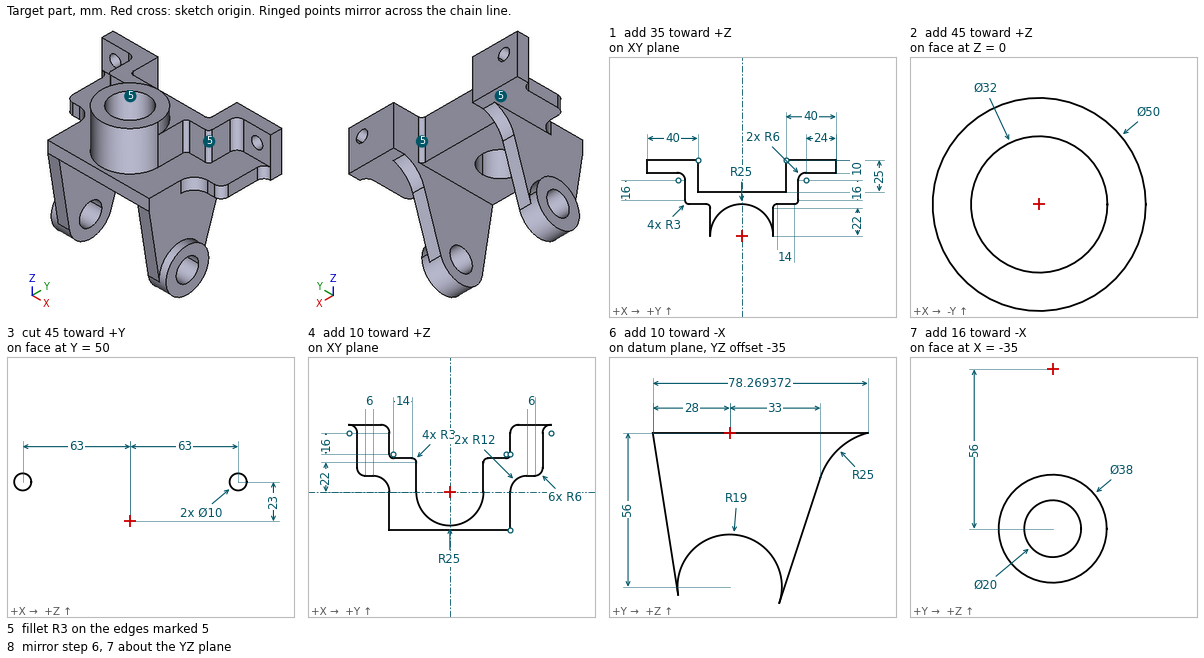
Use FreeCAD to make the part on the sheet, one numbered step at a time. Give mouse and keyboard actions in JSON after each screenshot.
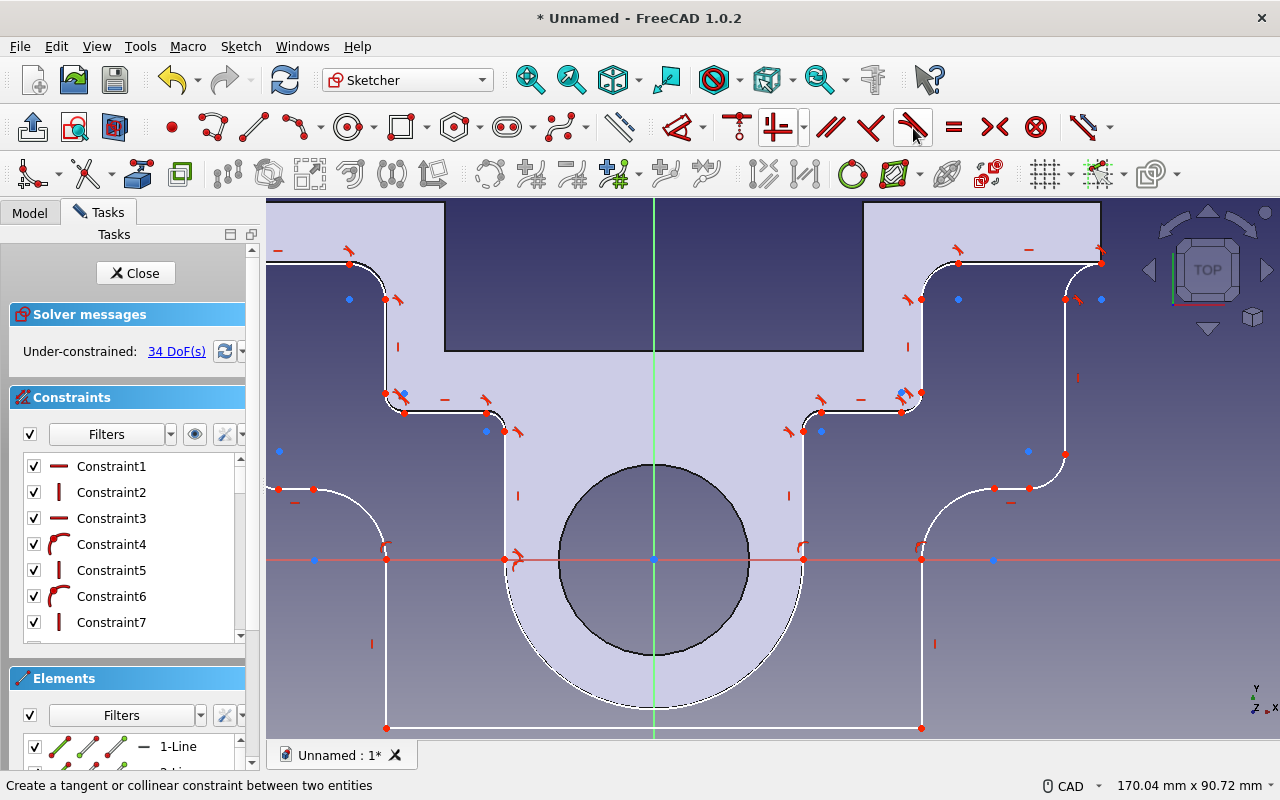
{"action": "left_click", "coordinate": [1065, 346]}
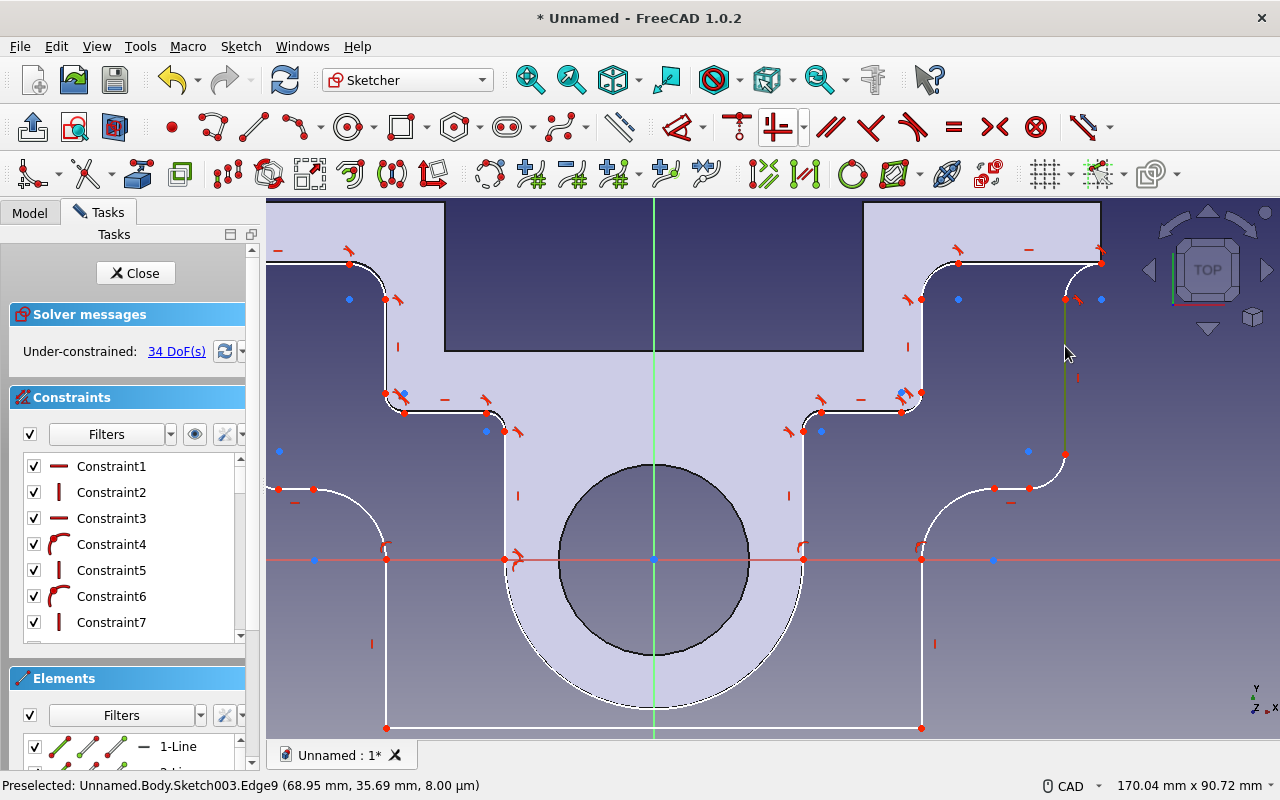
{"action": "left_click", "coordinate": [1045, 485]}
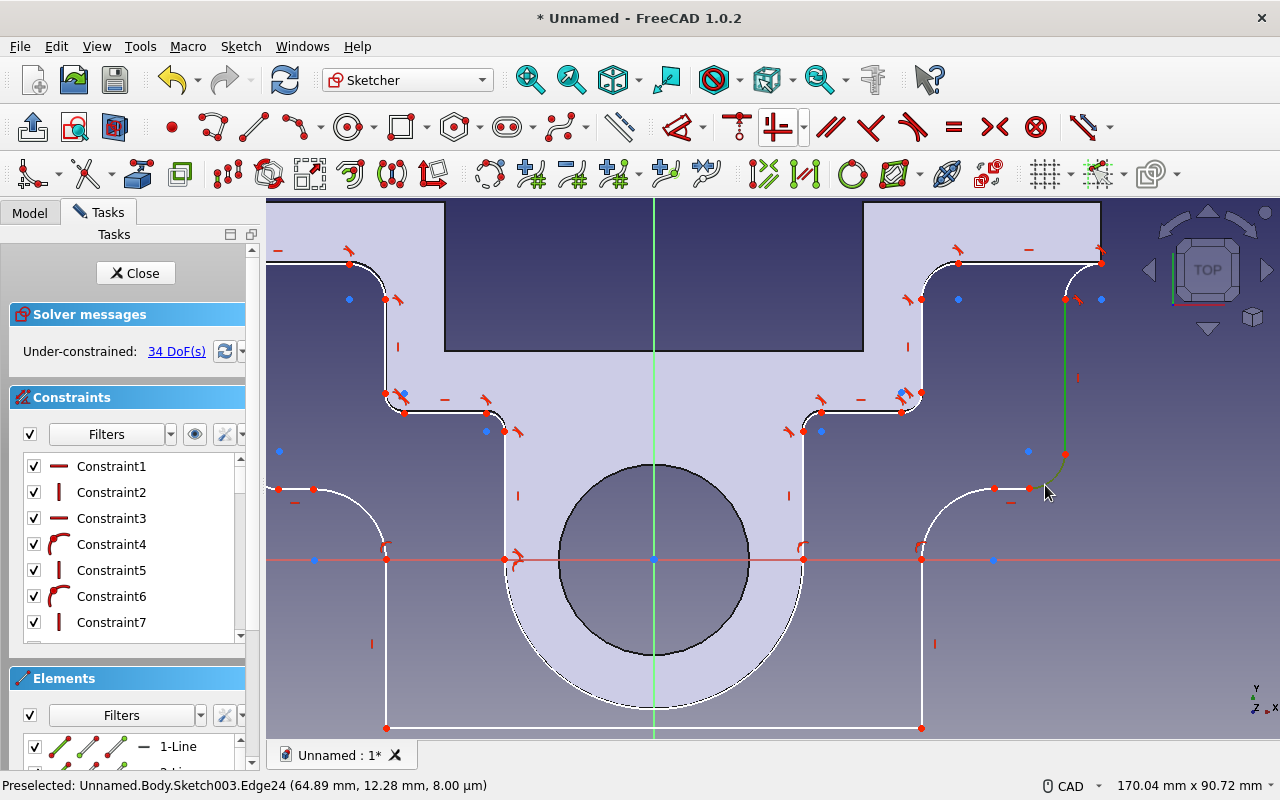
{"action": "left_click", "coordinate": [913, 128]}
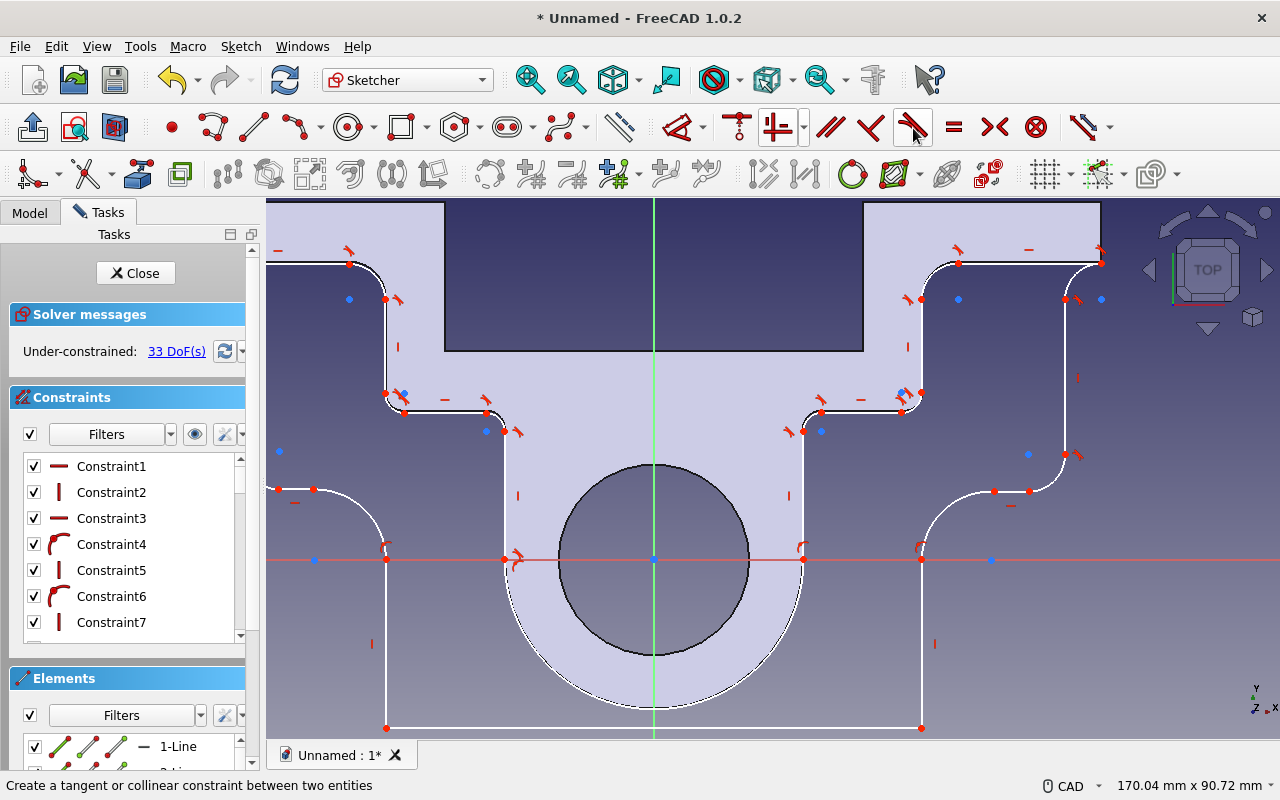
{"action": "scroll", "coordinate": [1019, 492], "scroll_direction": "up", "scroll_amount": 2}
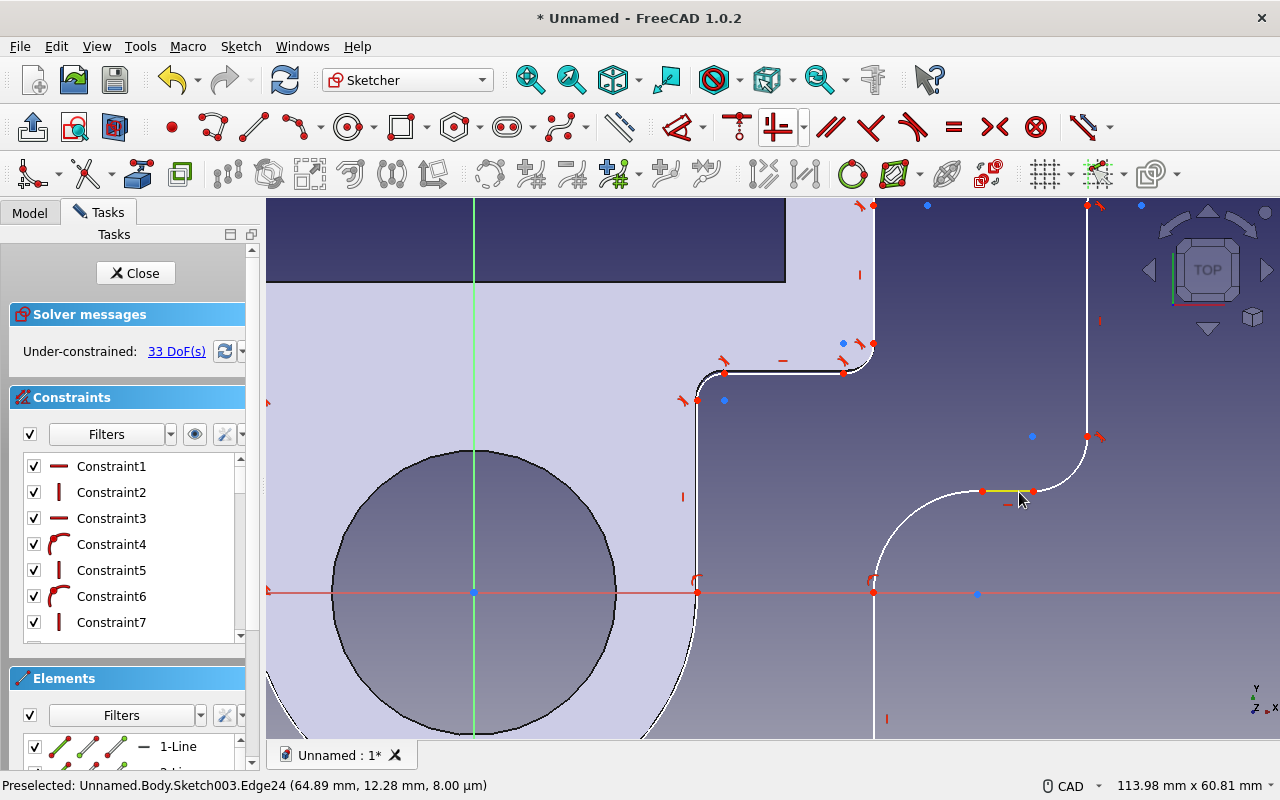
{"action": "left_click", "coordinate": [1018, 491]}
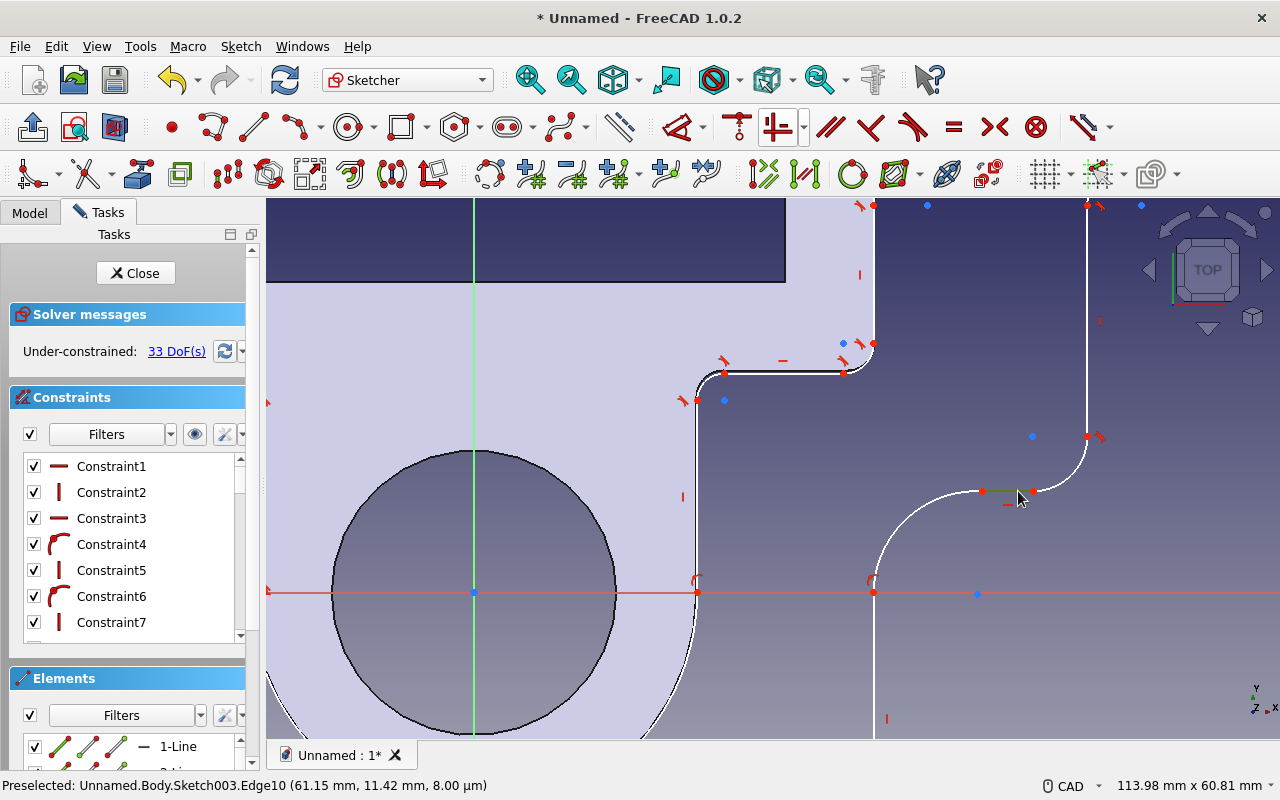
{"action": "left_click", "coordinate": [1058, 485]}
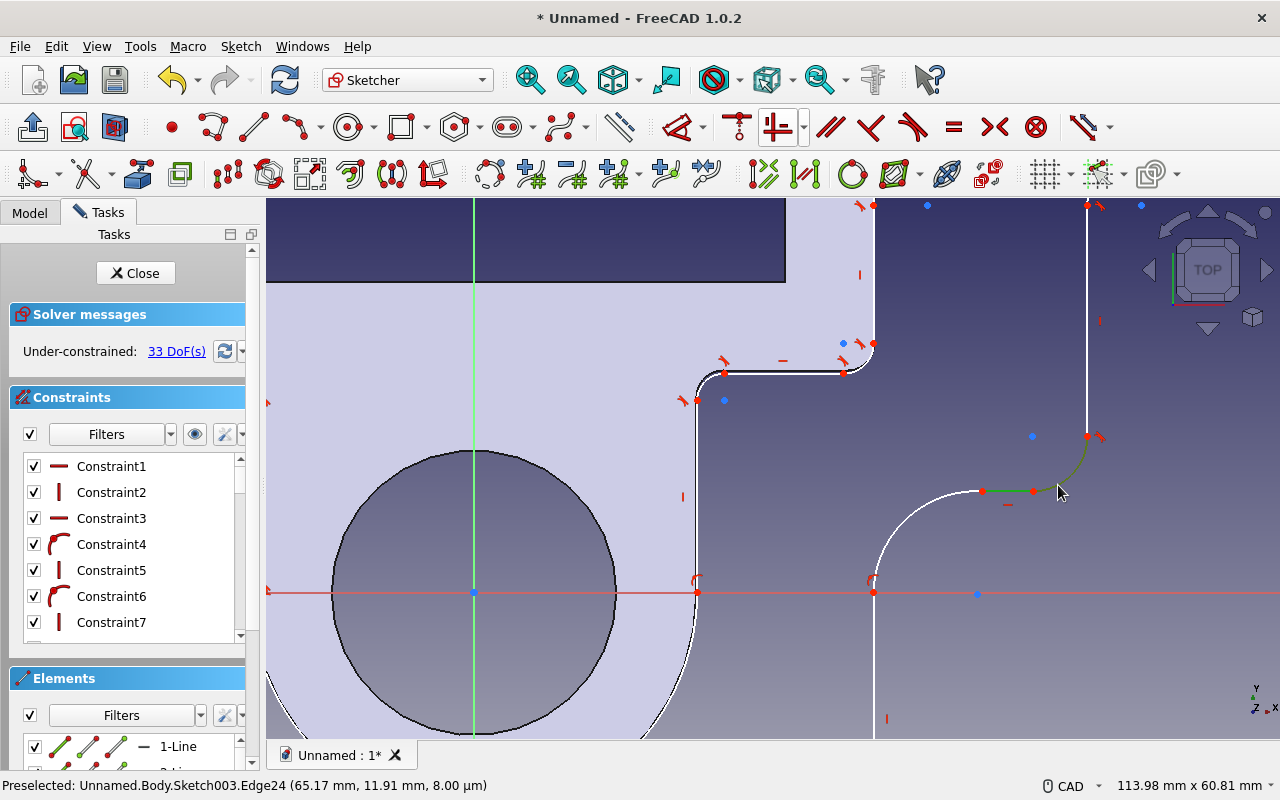
{"action": "left_click", "coordinate": [913, 128]}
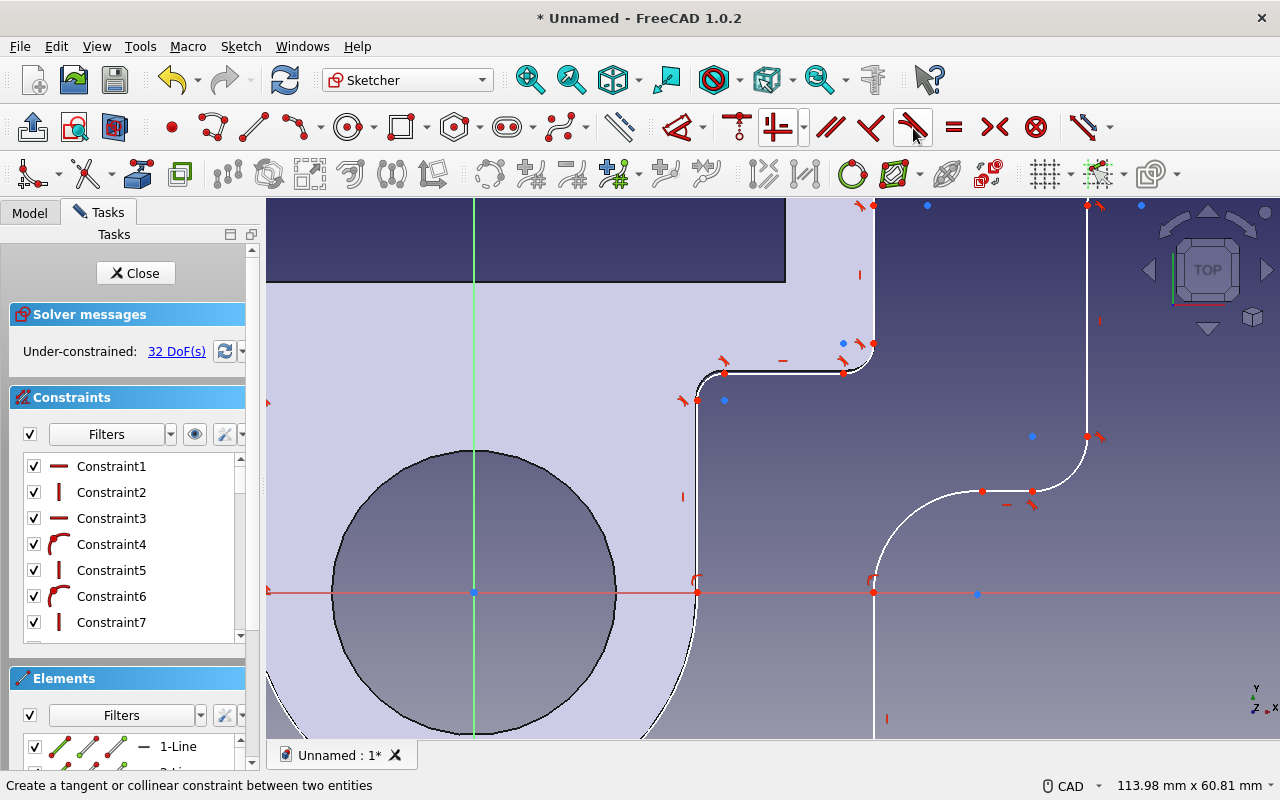
{"action": "left_click", "coordinate": [1017, 491]}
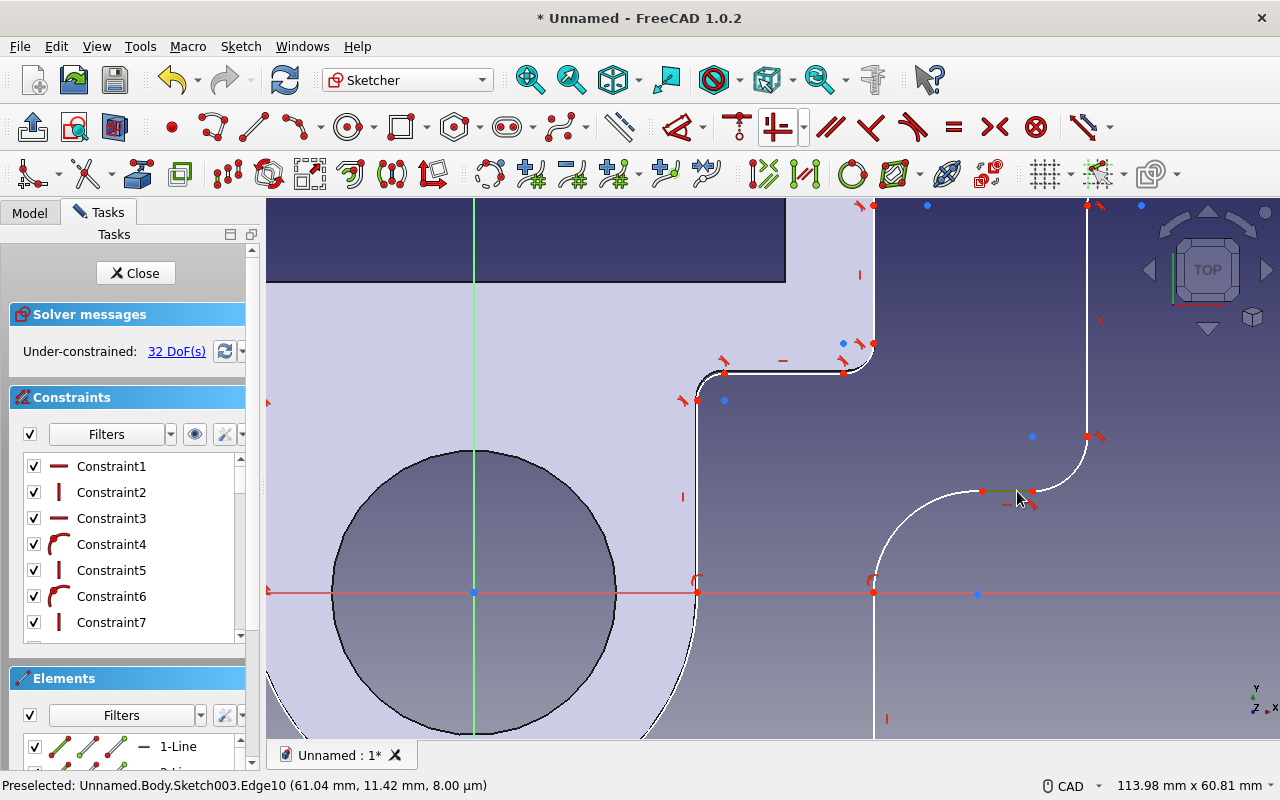
{"action": "left_click", "coordinate": [934, 501]}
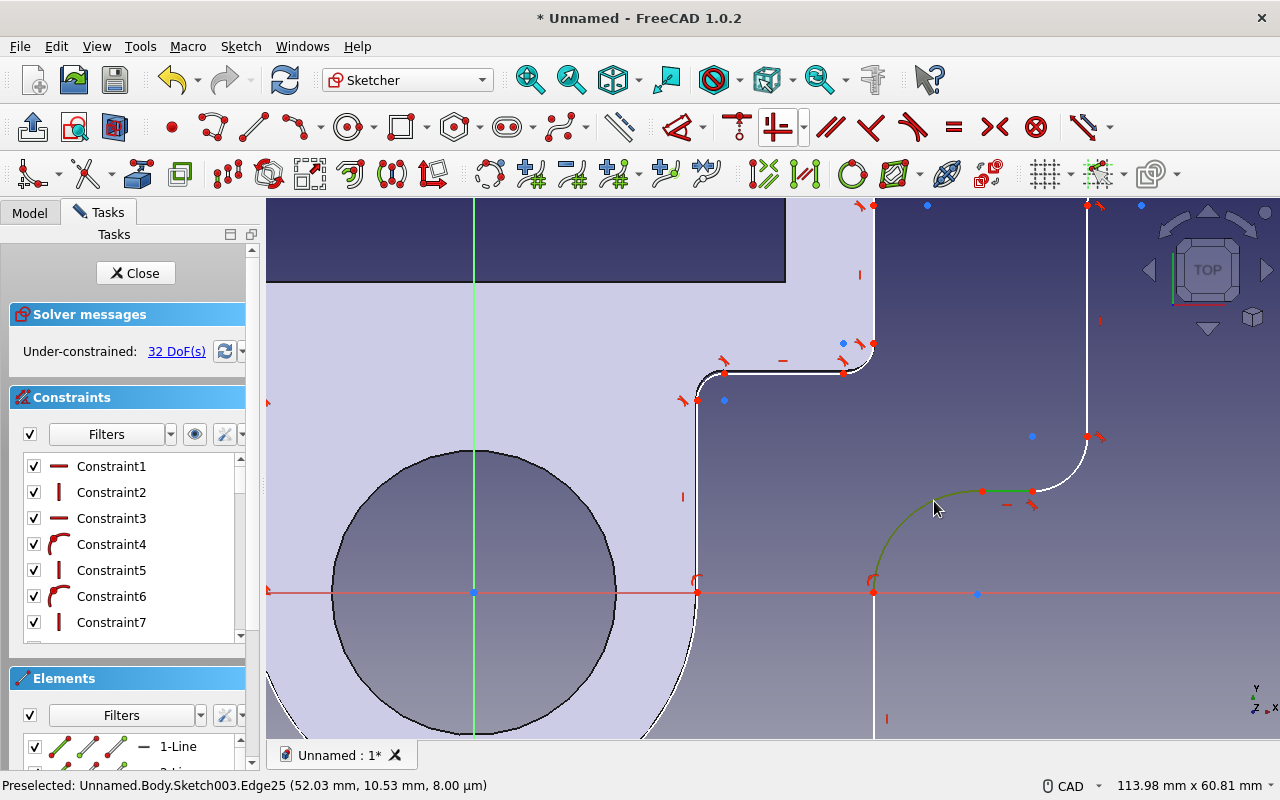
{"action": "left_click", "coordinate": [913, 128]}